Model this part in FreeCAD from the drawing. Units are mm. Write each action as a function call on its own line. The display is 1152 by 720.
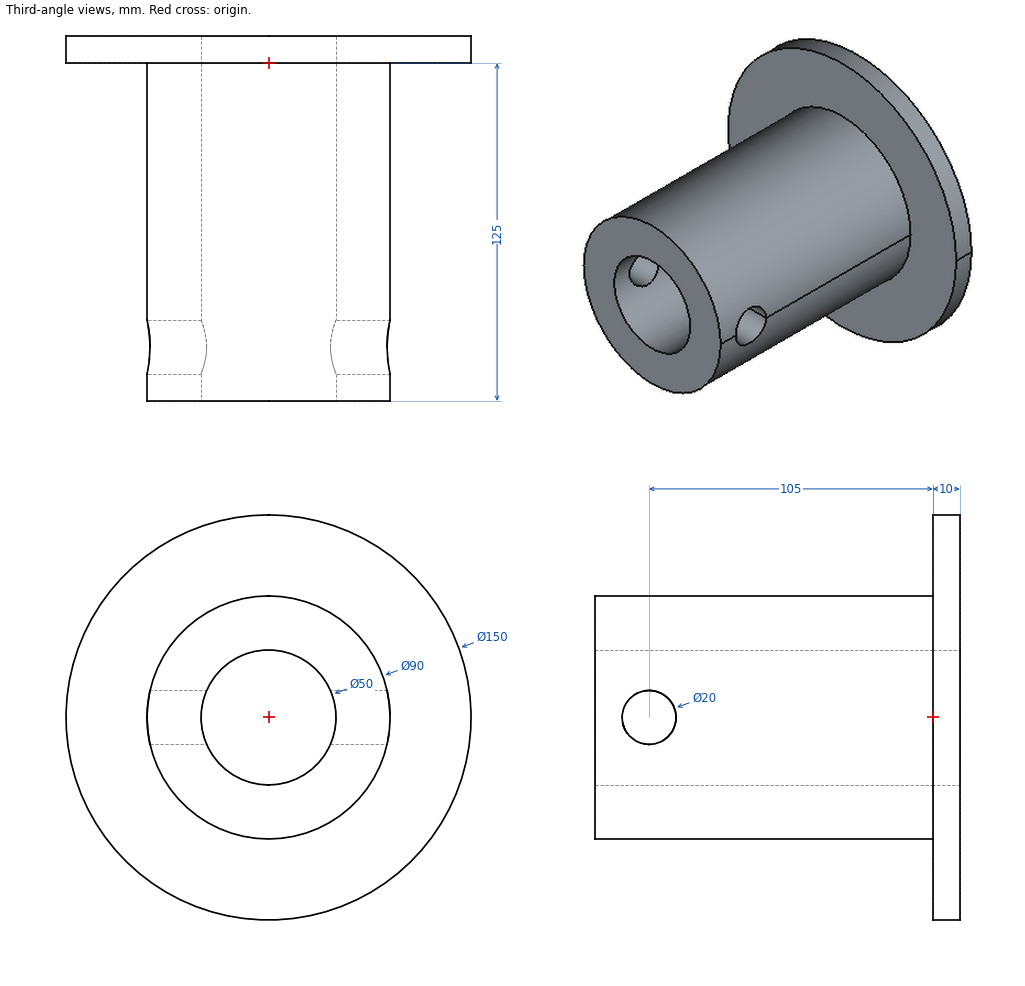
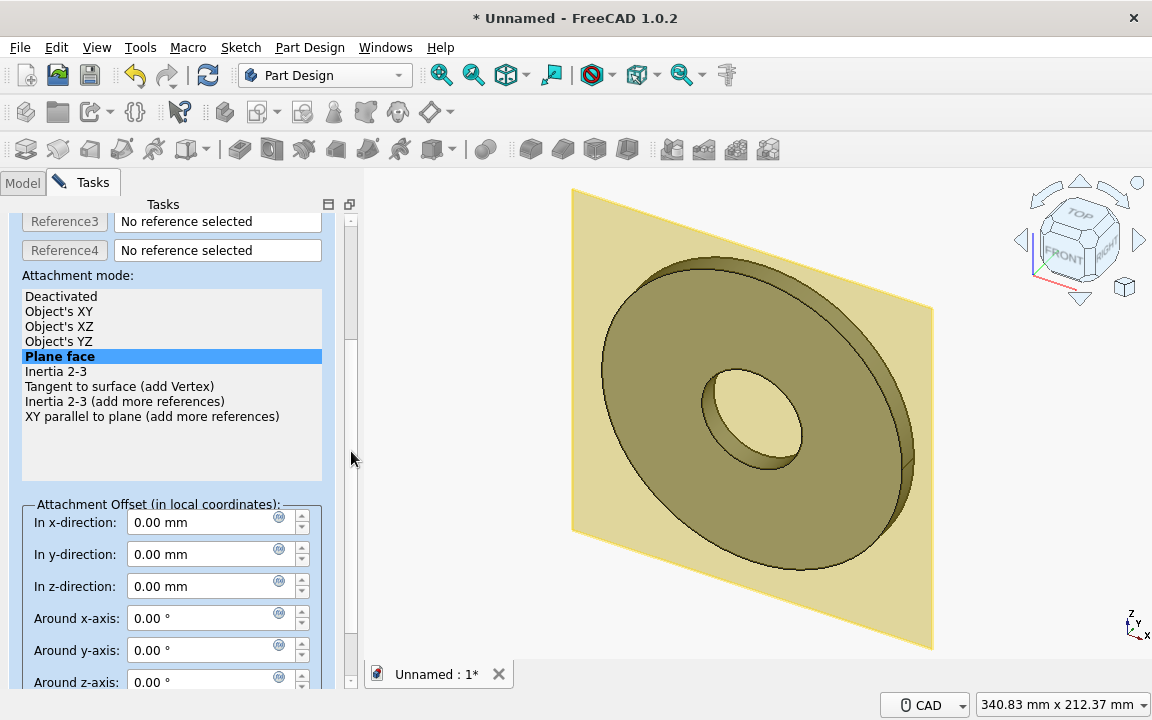
triple_click(210, 586)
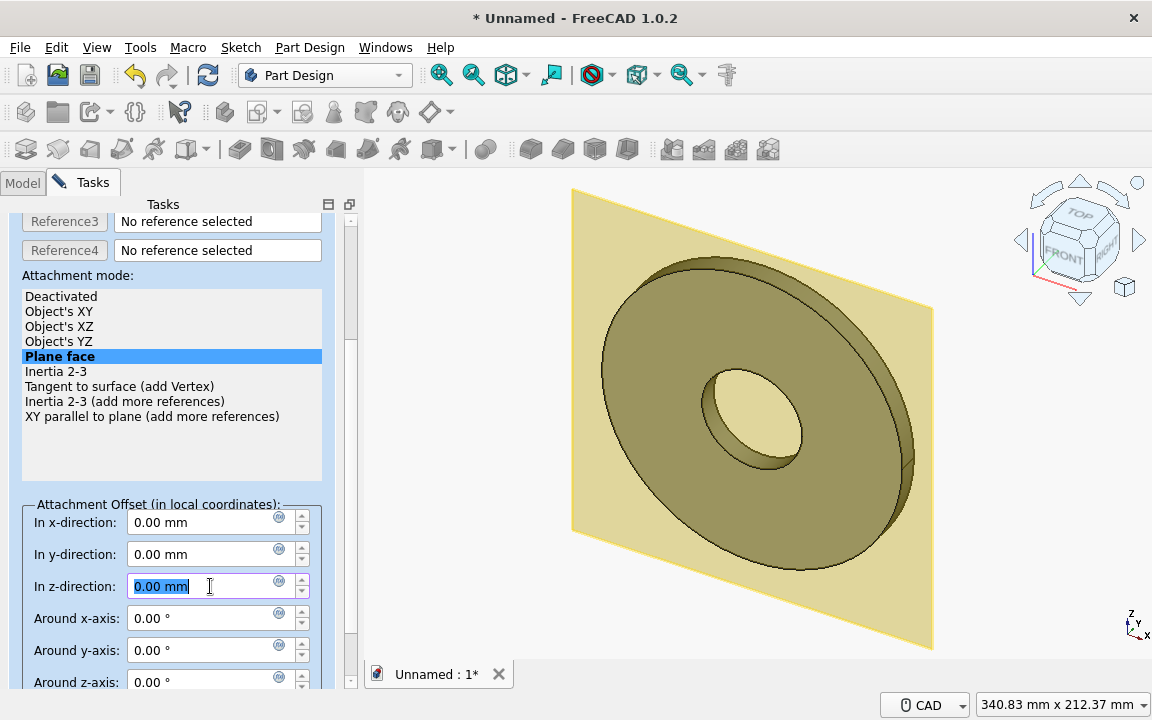
text(125)
key(Tab)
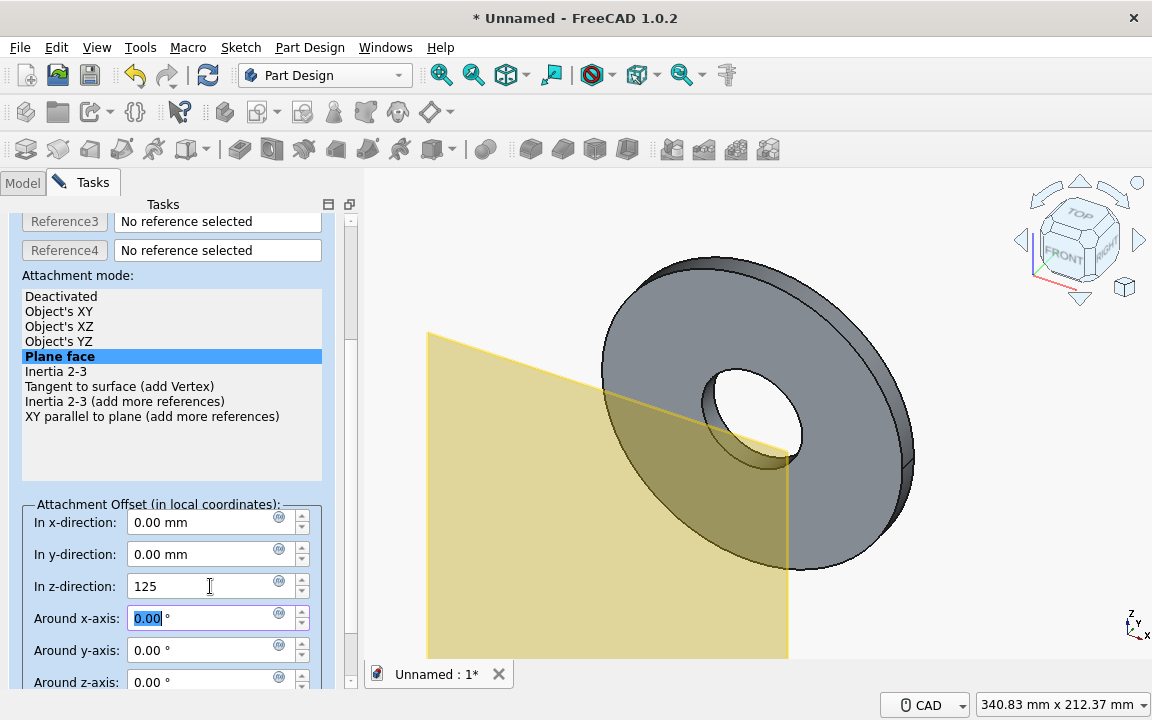
scroll(351, 451, up, 4)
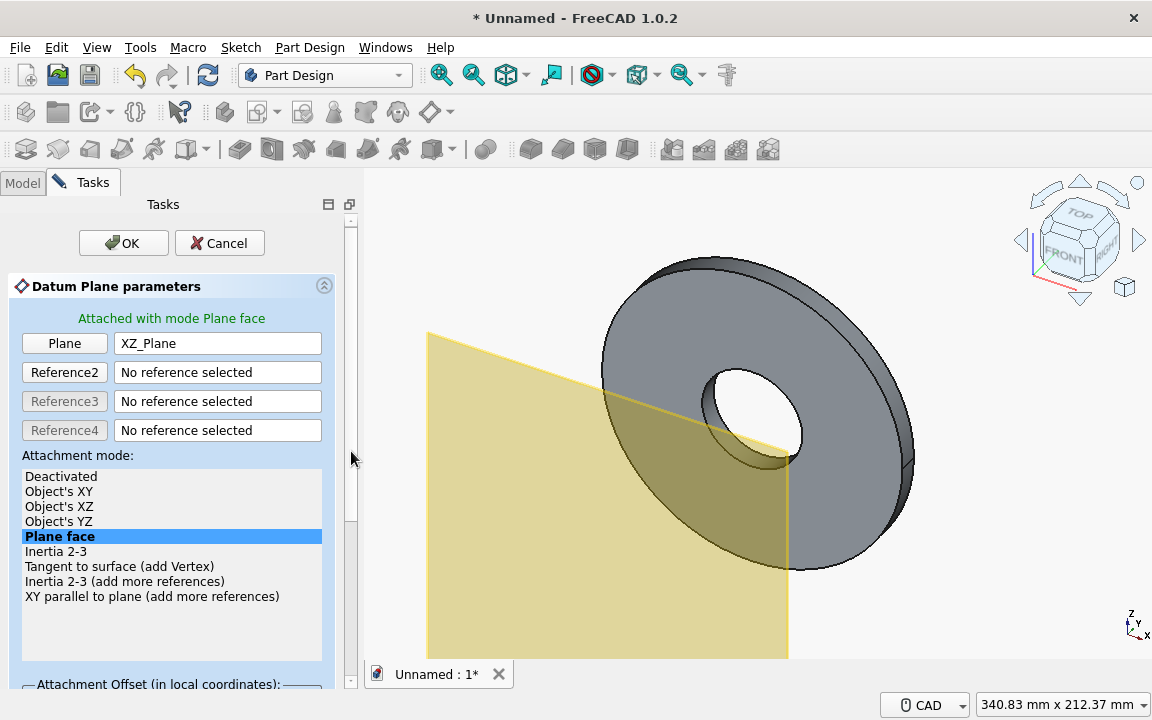
click(124, 243)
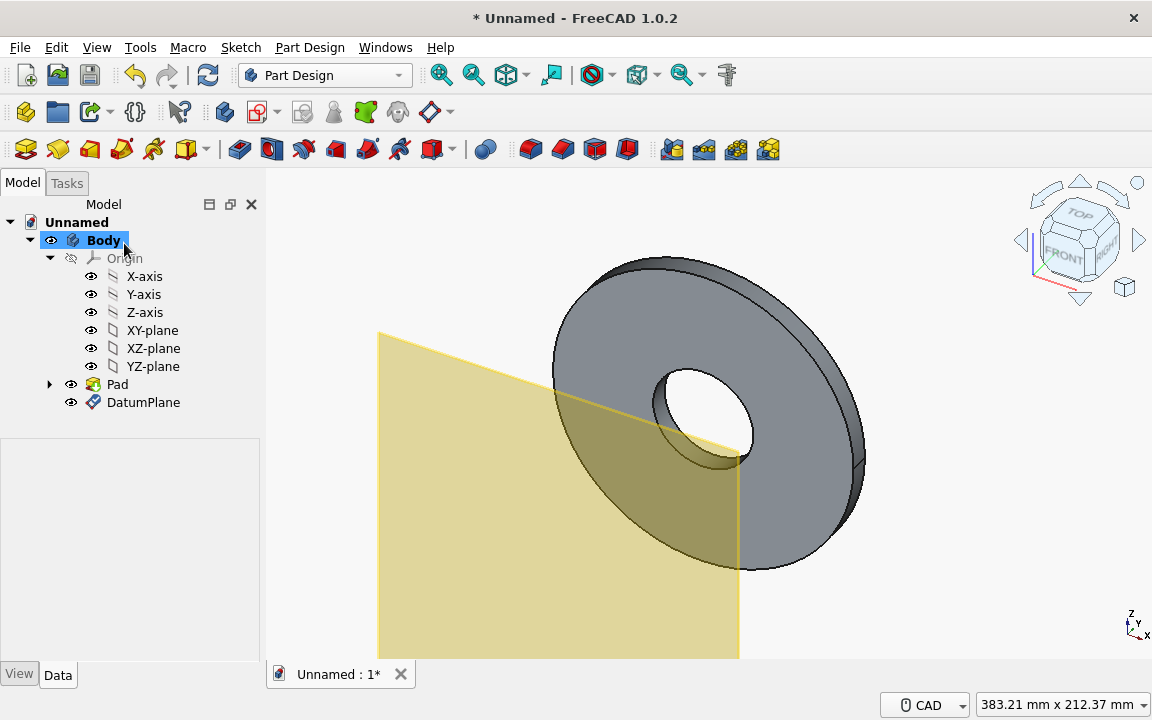
click(116, 402)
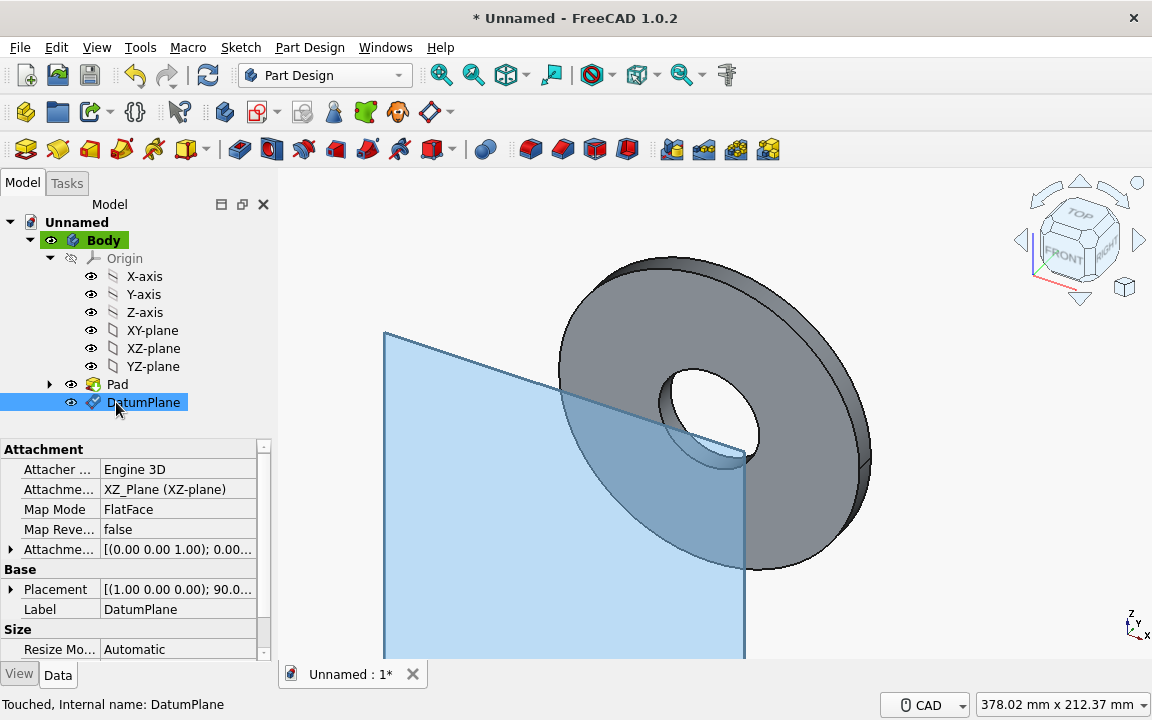
click(258, 112)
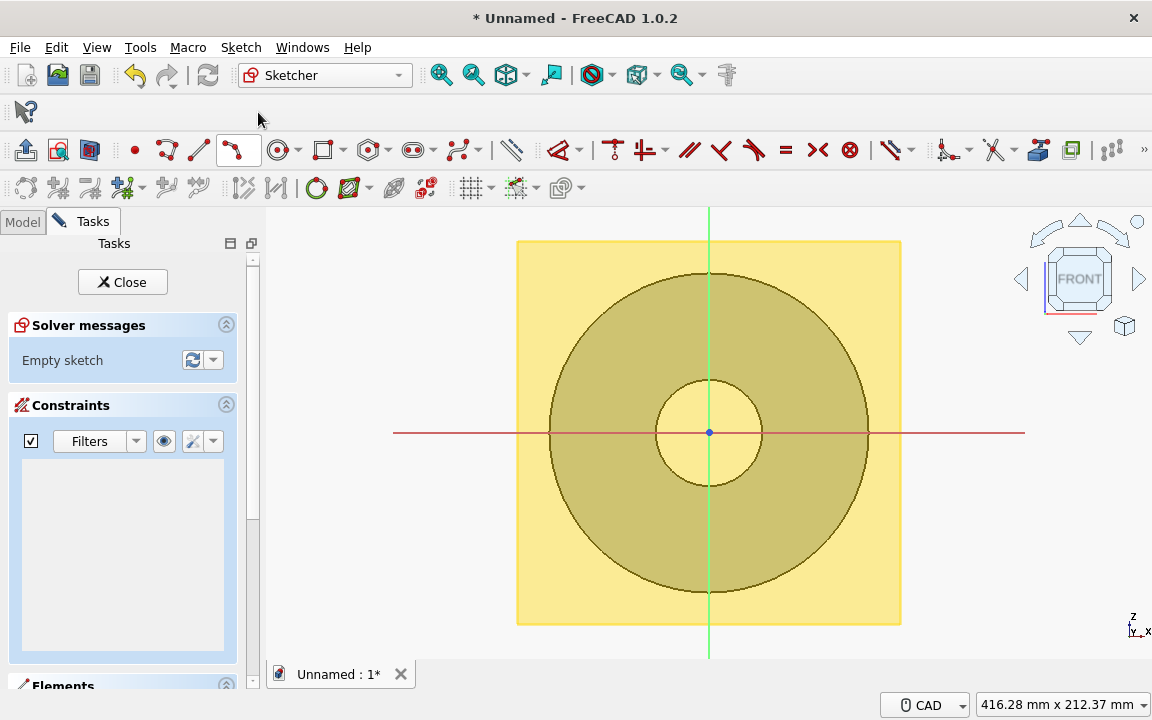
scroll(848, 433, up, 2)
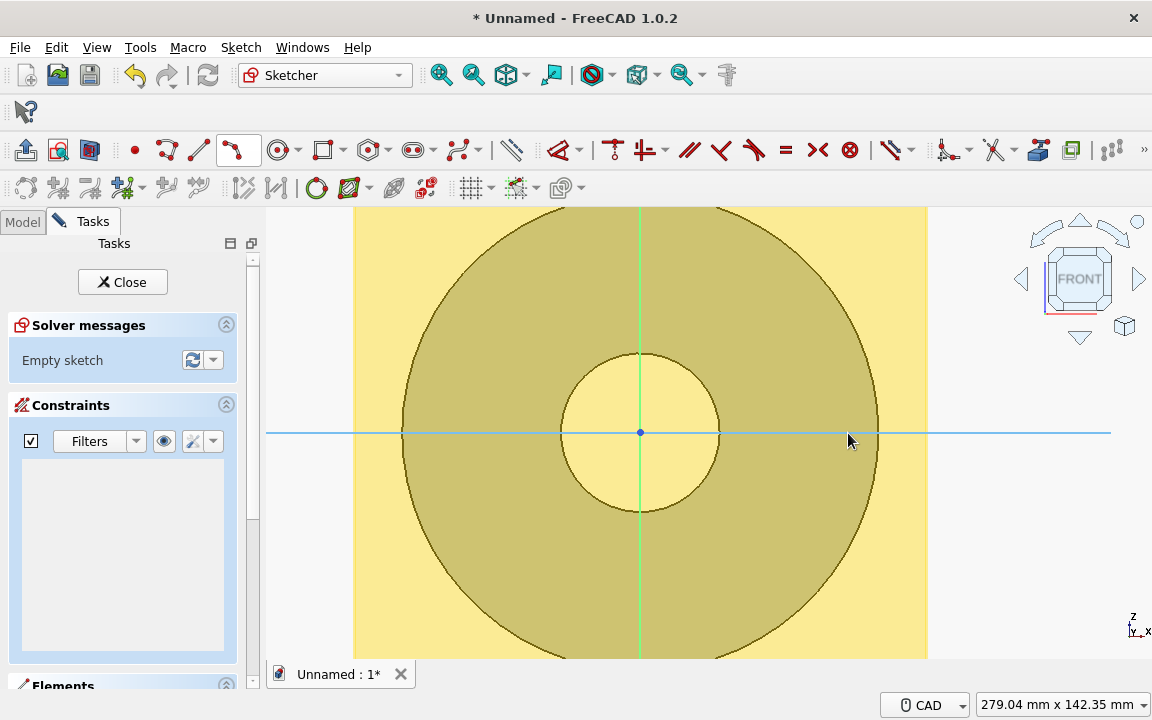
click(278, 150)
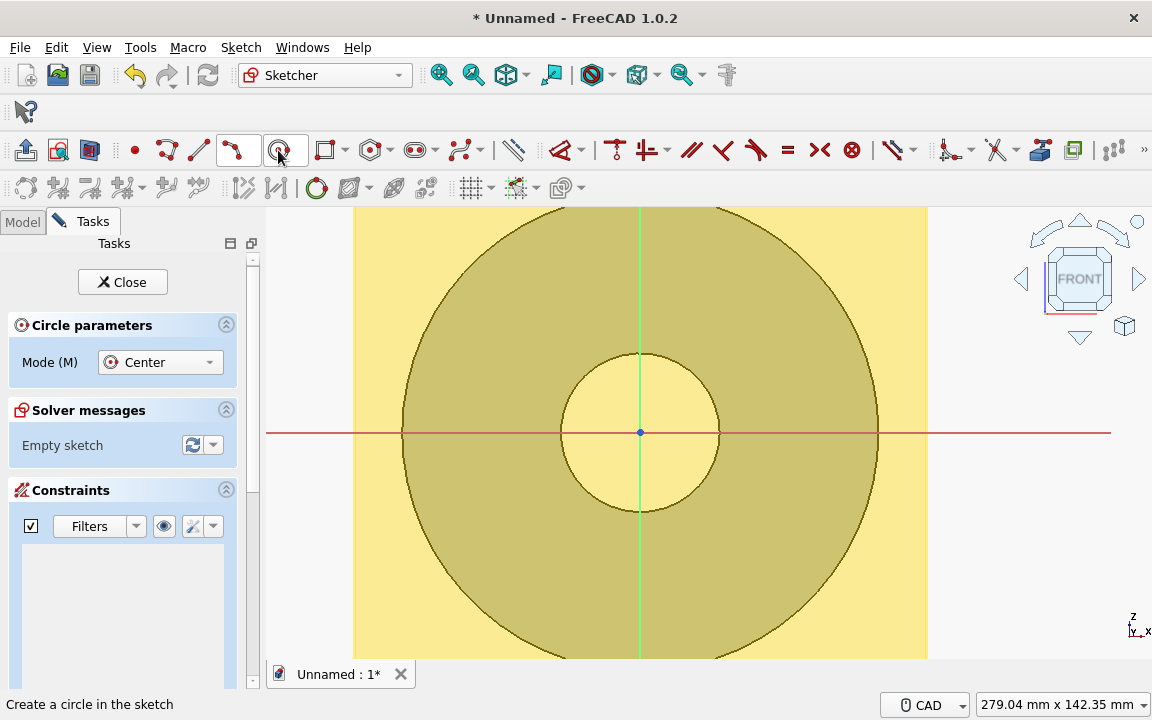
click(640, 433)
click(741, 332)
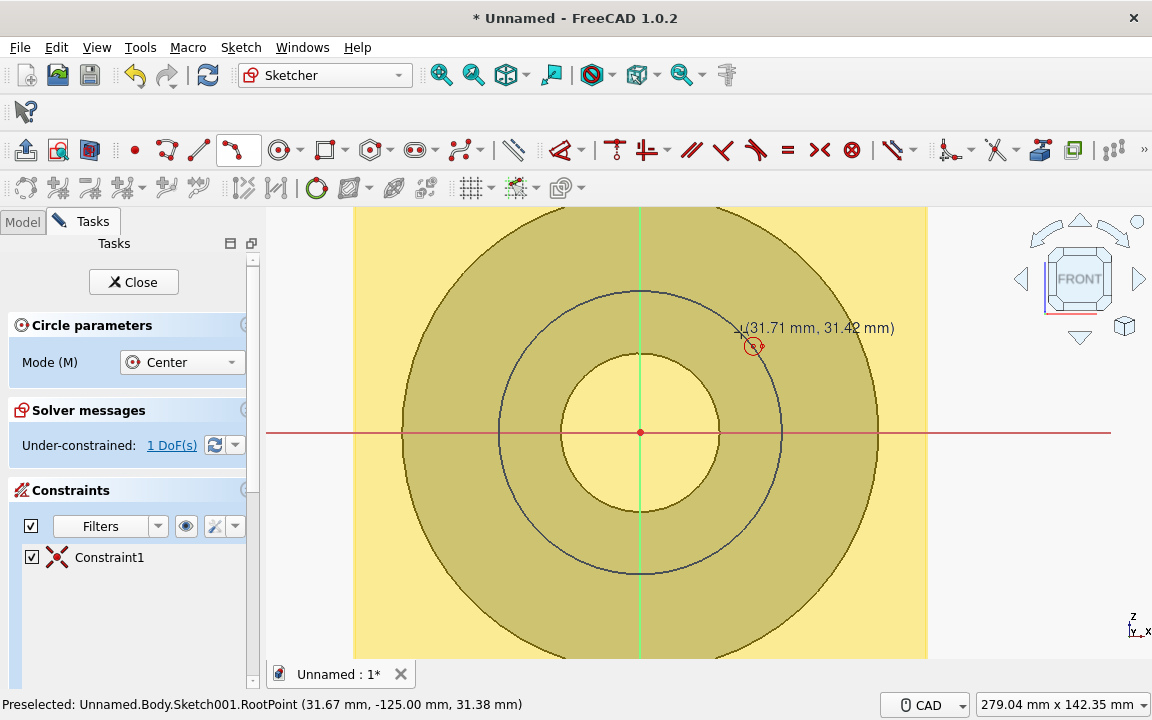
click(640, 433)
click(696, 377)
key(Escape)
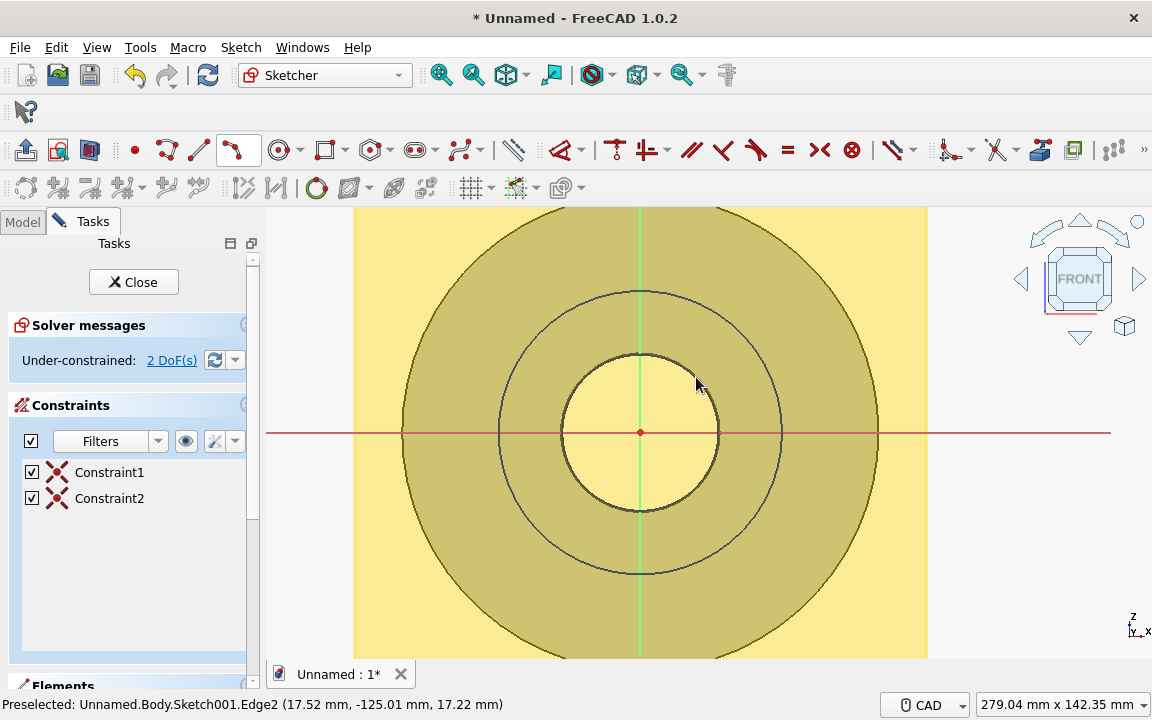
click(560, 150)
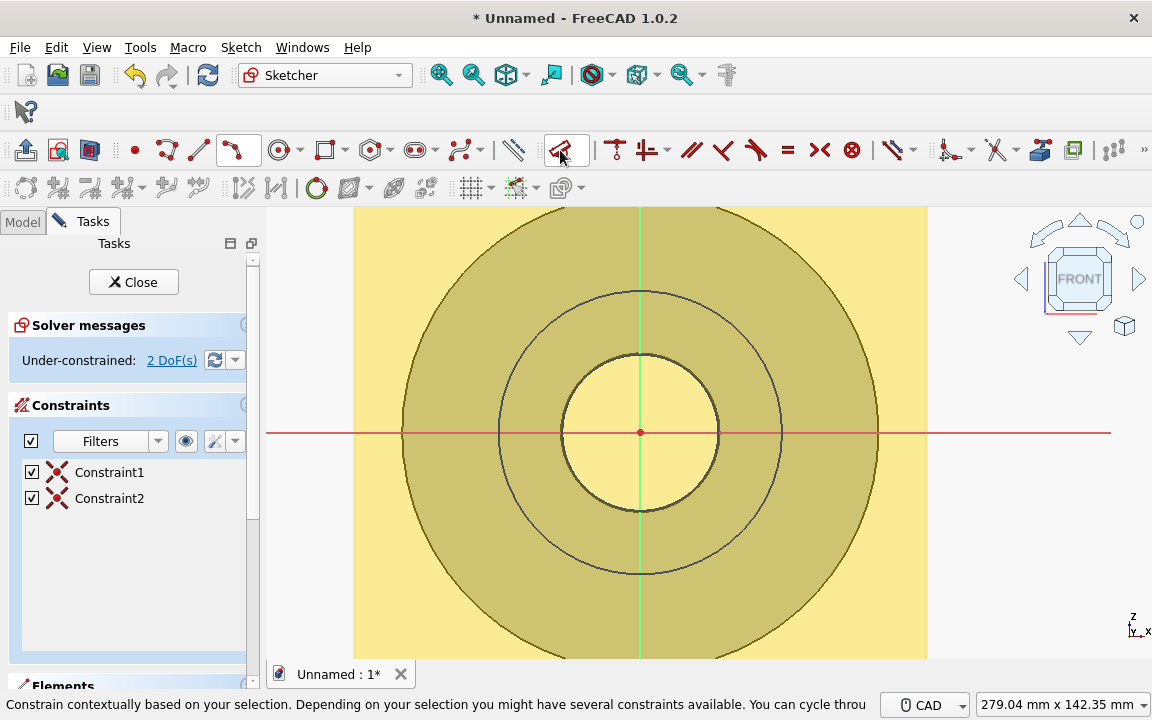
click(740, 332)
click(763, 309)